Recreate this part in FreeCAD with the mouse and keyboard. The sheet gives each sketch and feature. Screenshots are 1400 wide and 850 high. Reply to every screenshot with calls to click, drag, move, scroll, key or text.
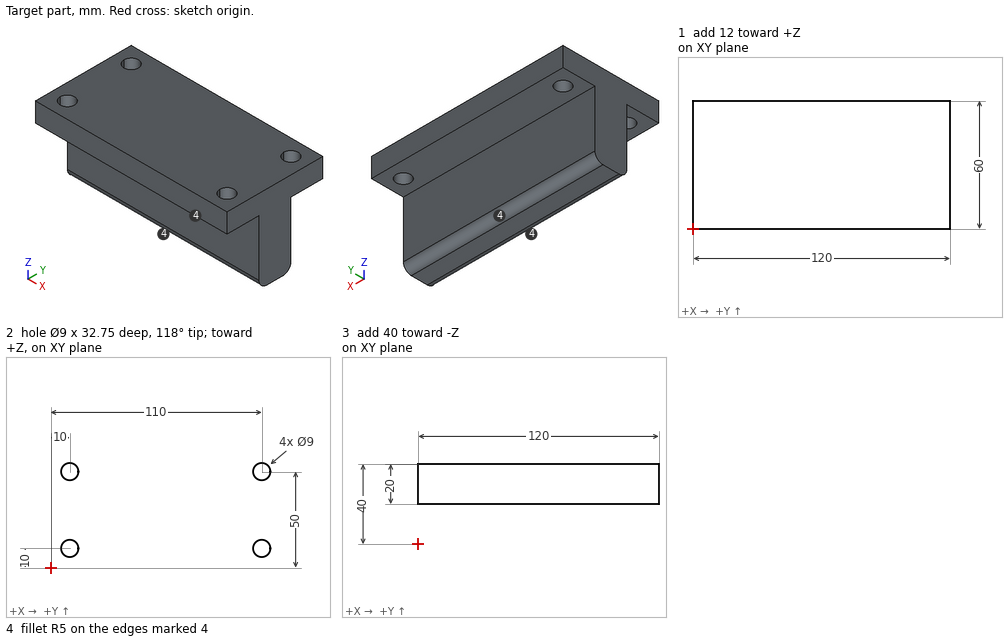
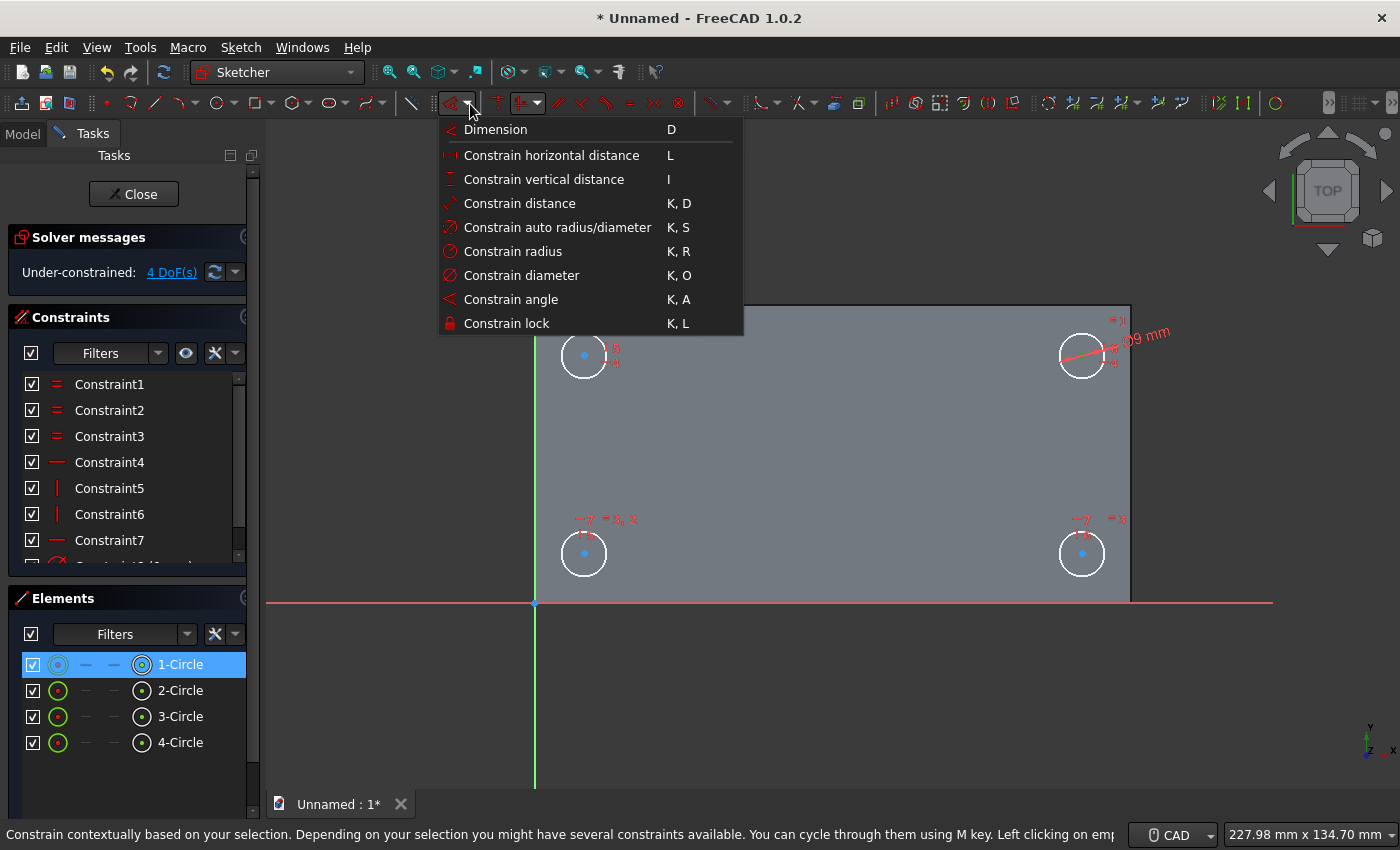
click(591, 179)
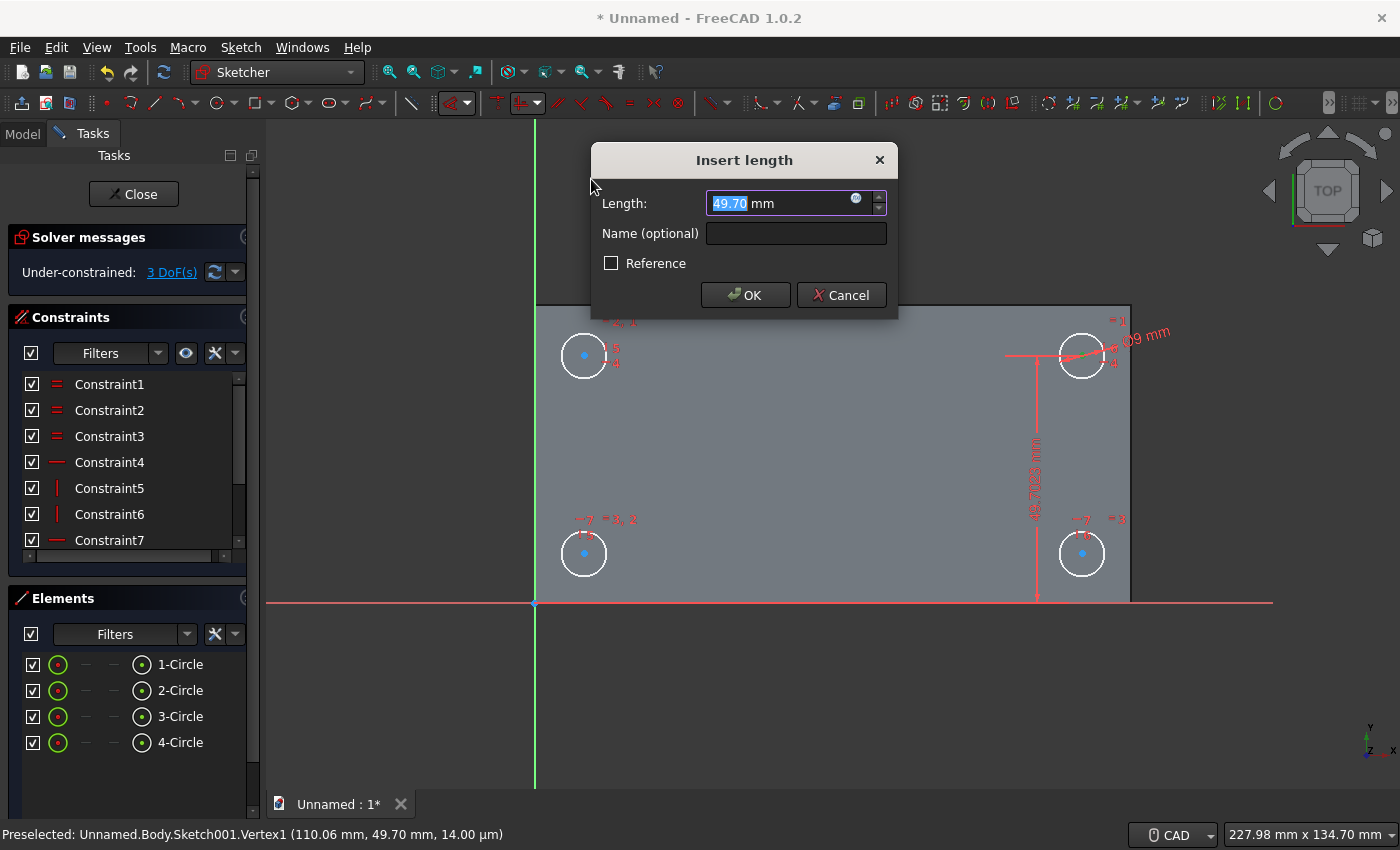
text(50)
key(Return)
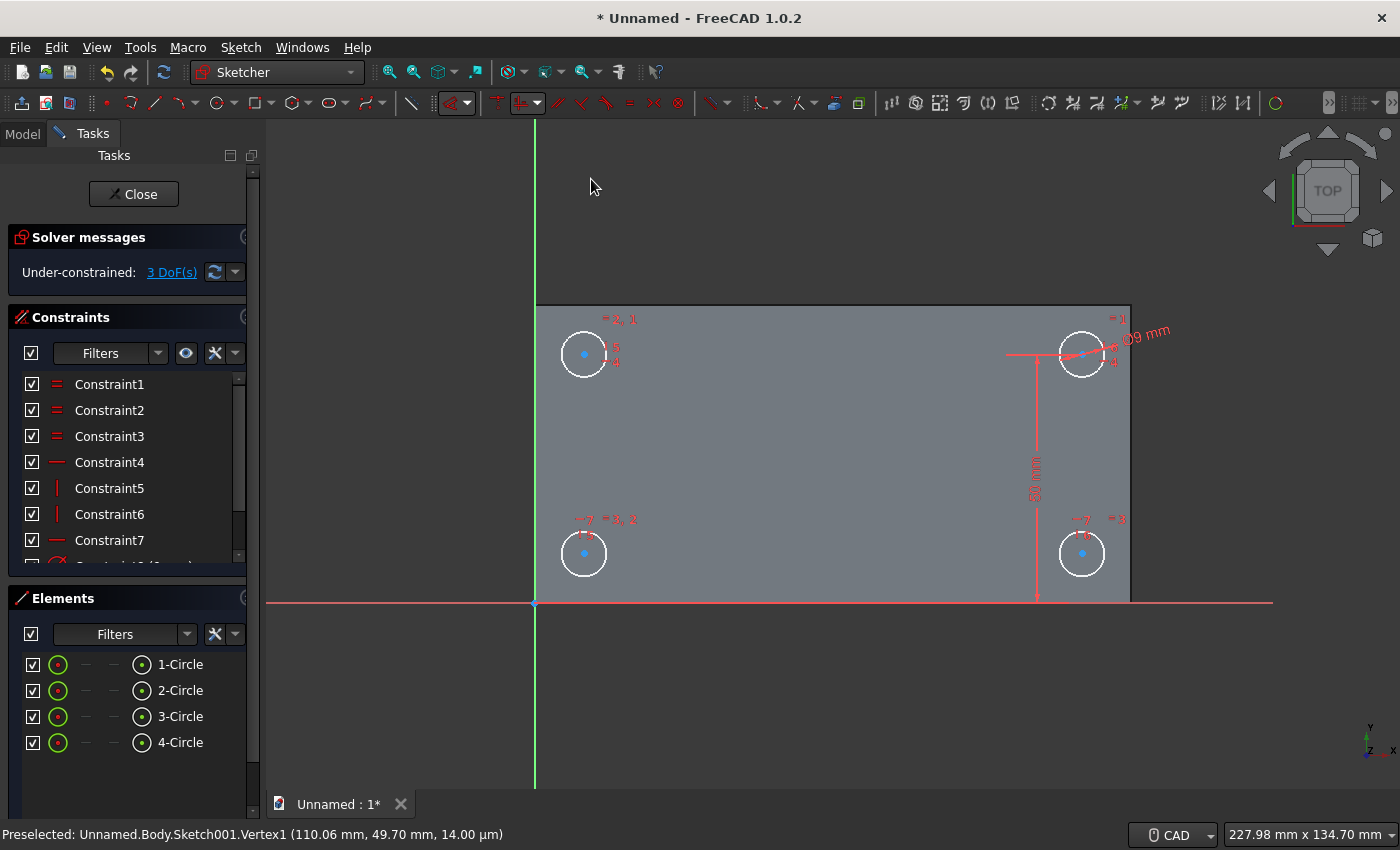
click(584, 355)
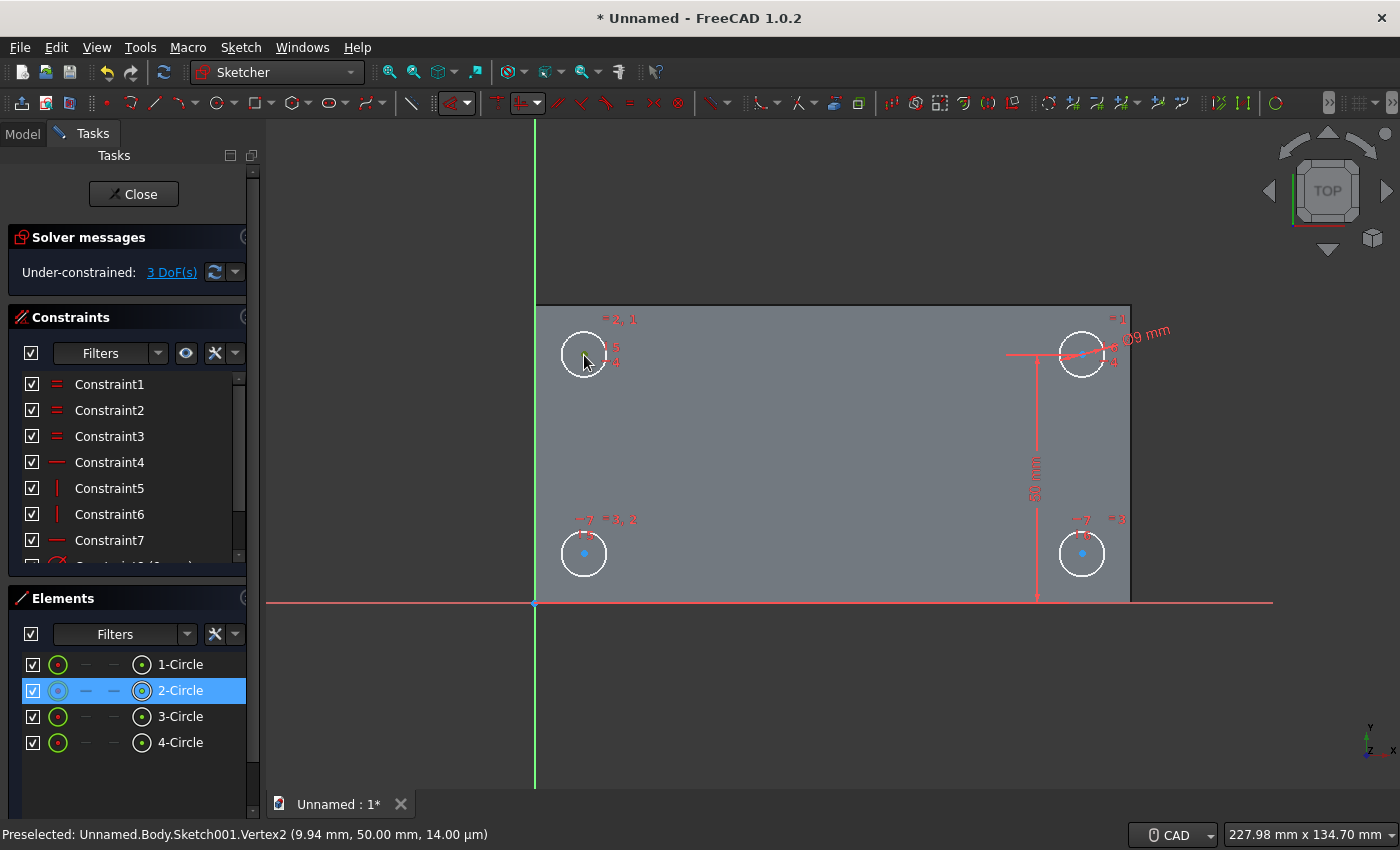
click(470, 104)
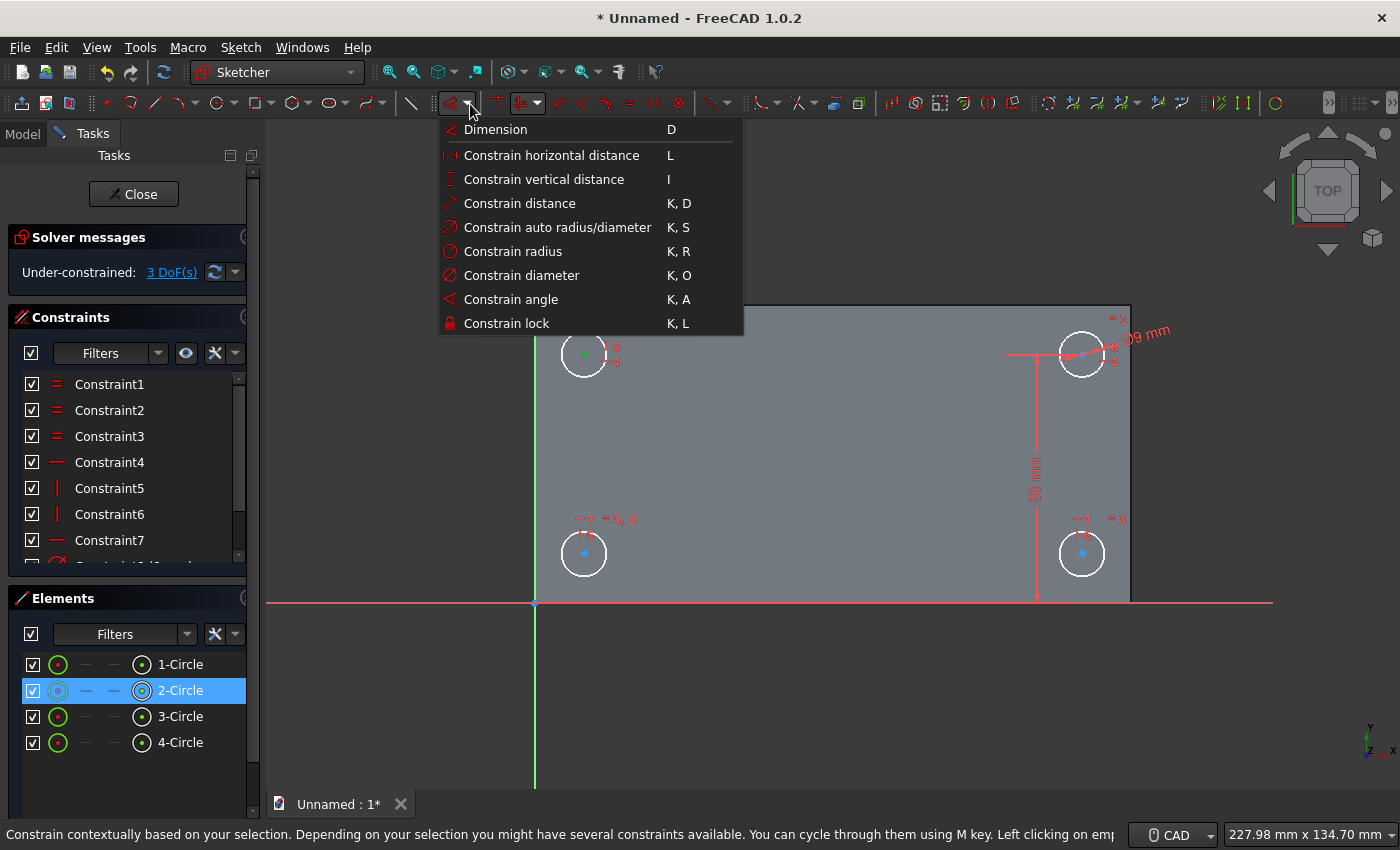
click(591, 155)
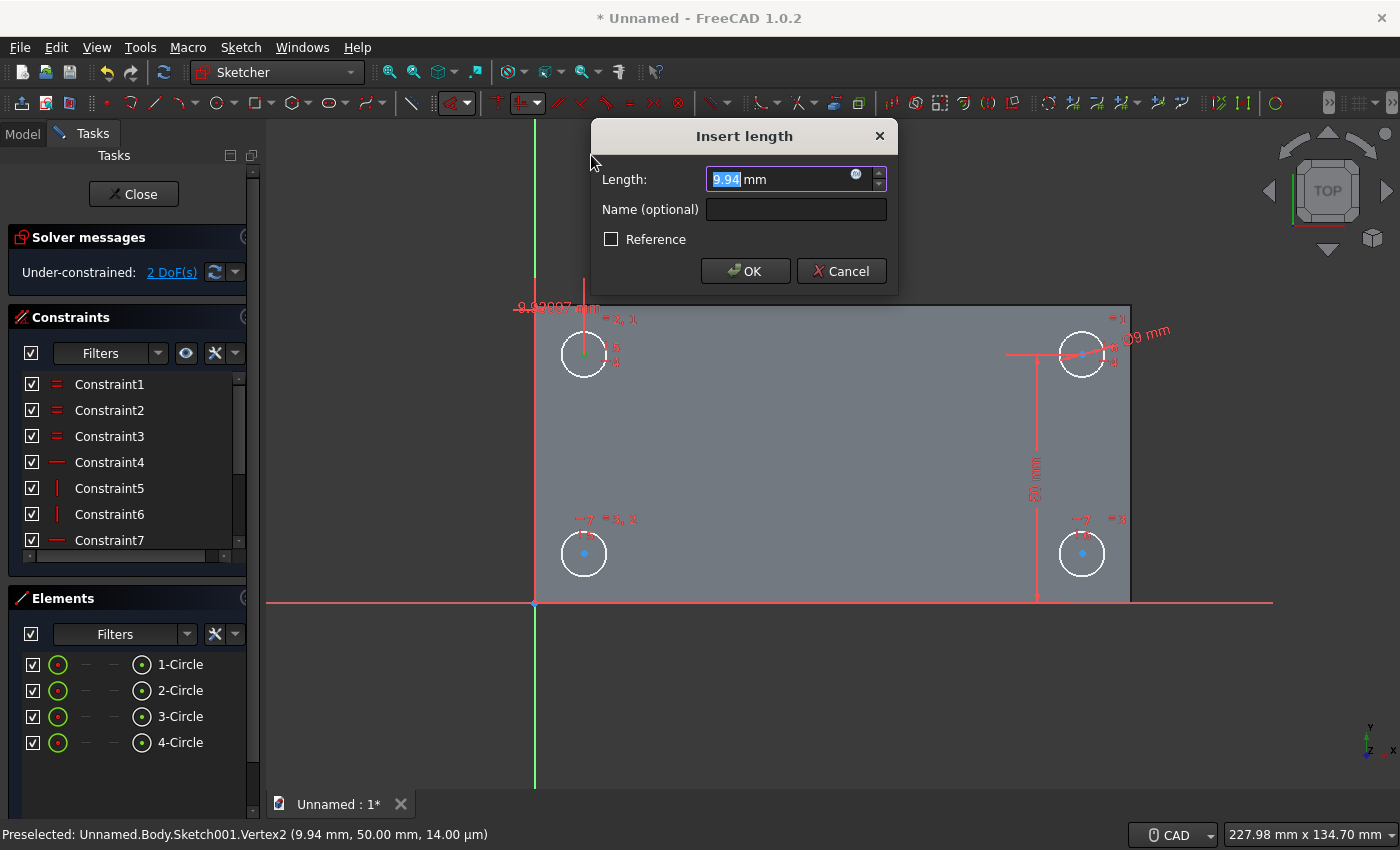
text(10)
key(Return)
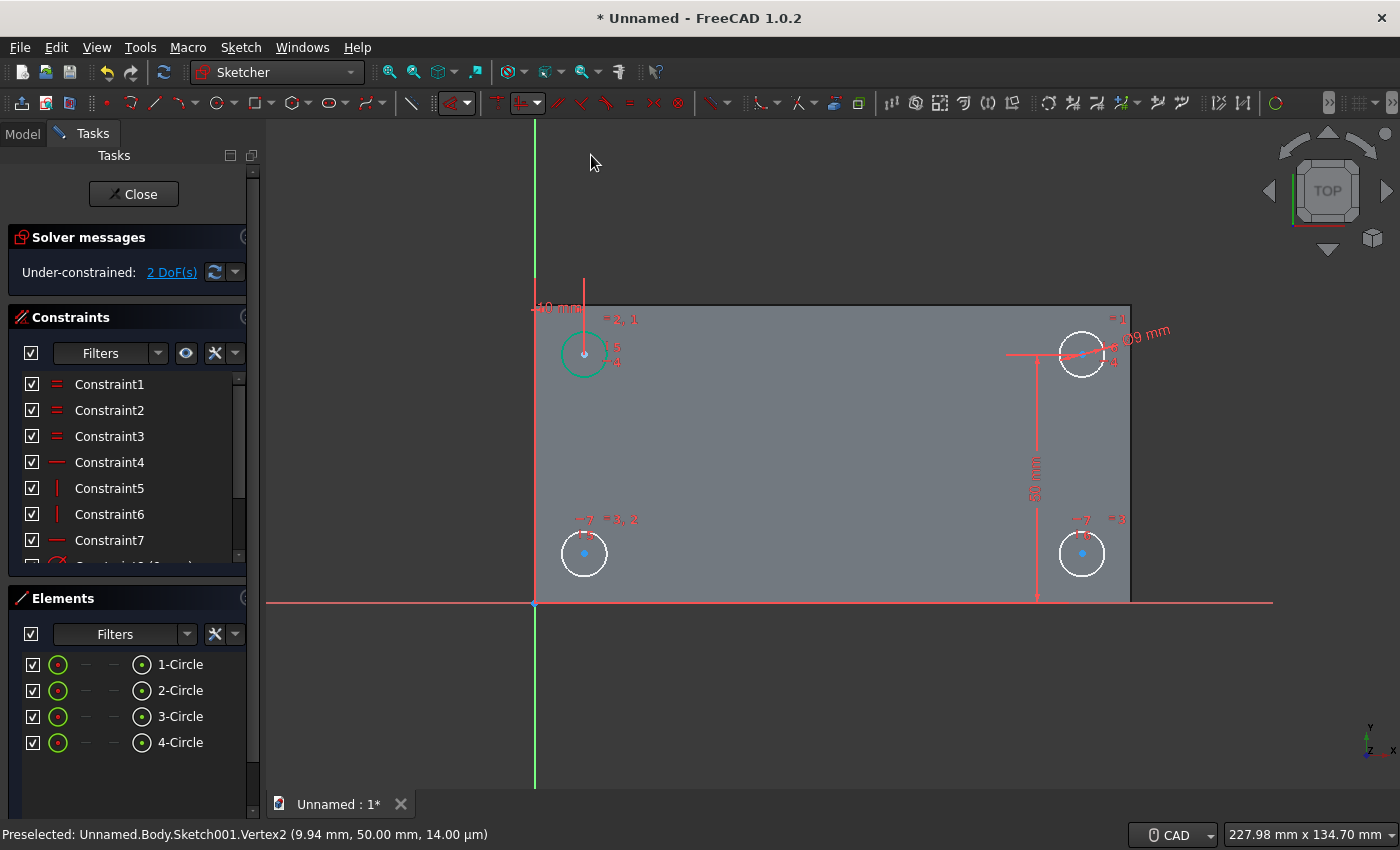
click(584, 554)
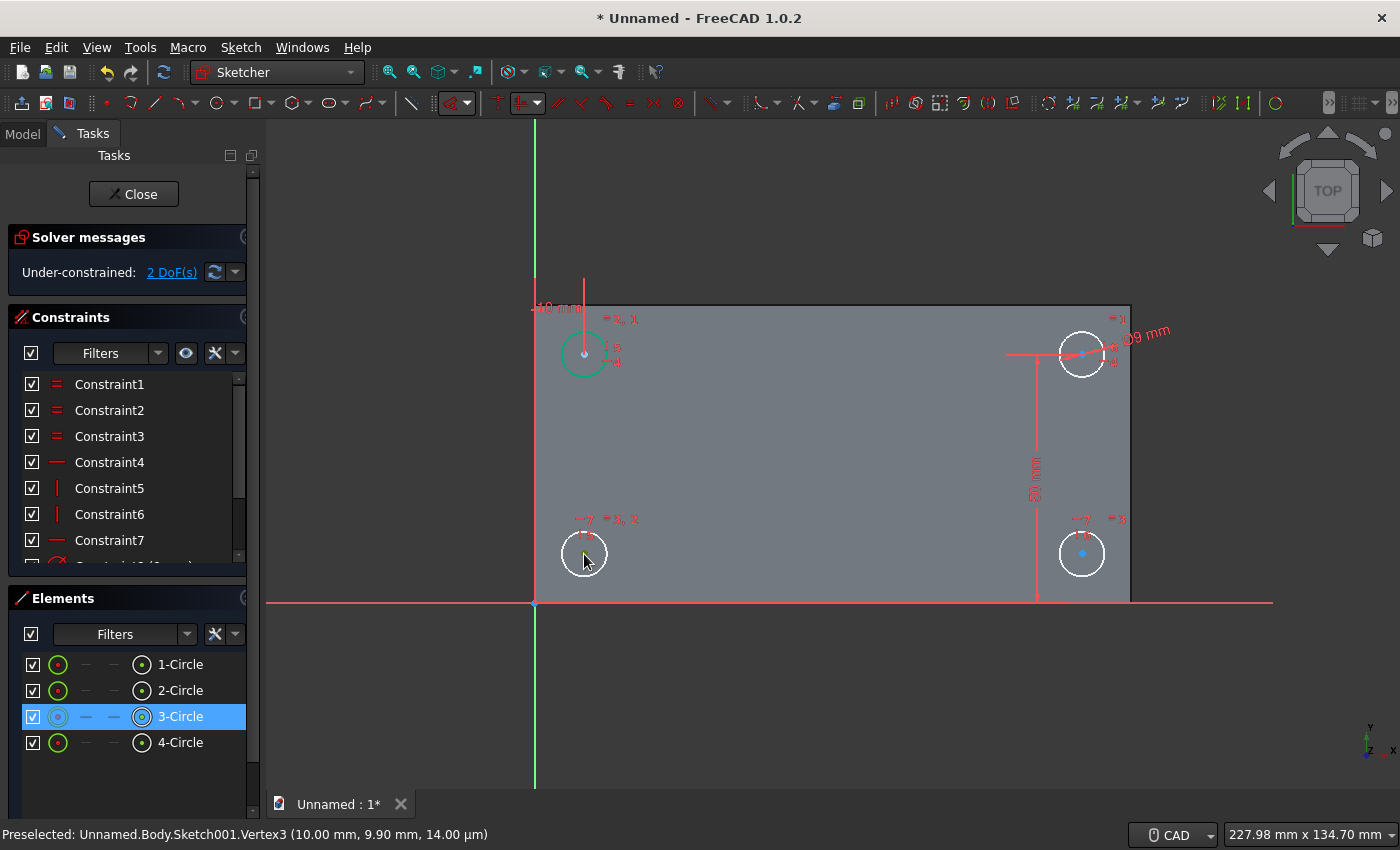
key(i)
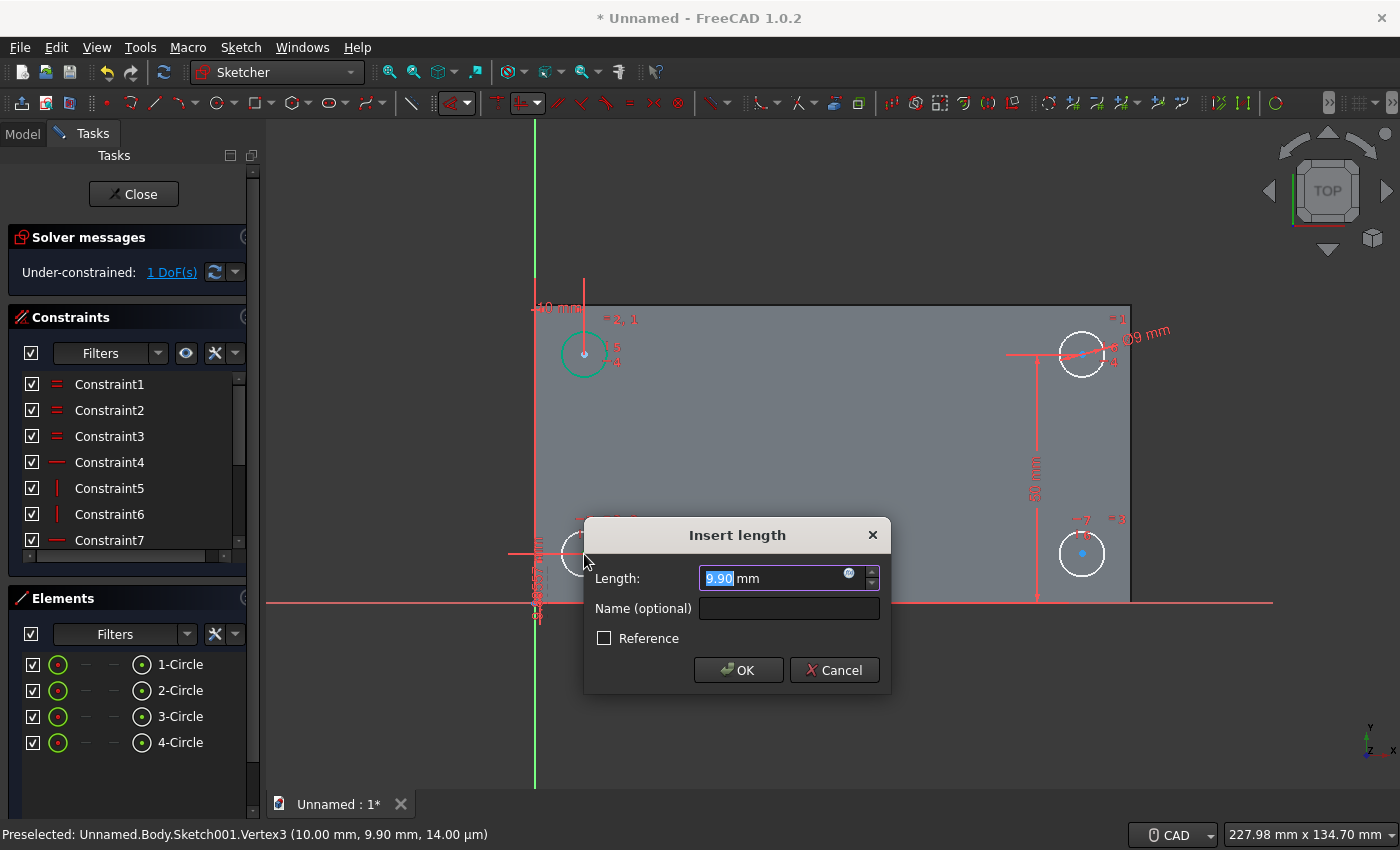
text(10)
key(Return)